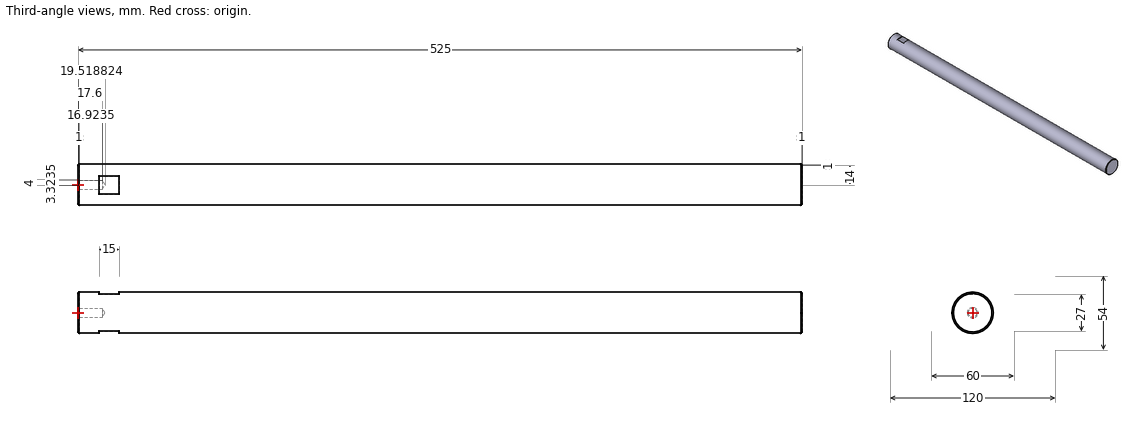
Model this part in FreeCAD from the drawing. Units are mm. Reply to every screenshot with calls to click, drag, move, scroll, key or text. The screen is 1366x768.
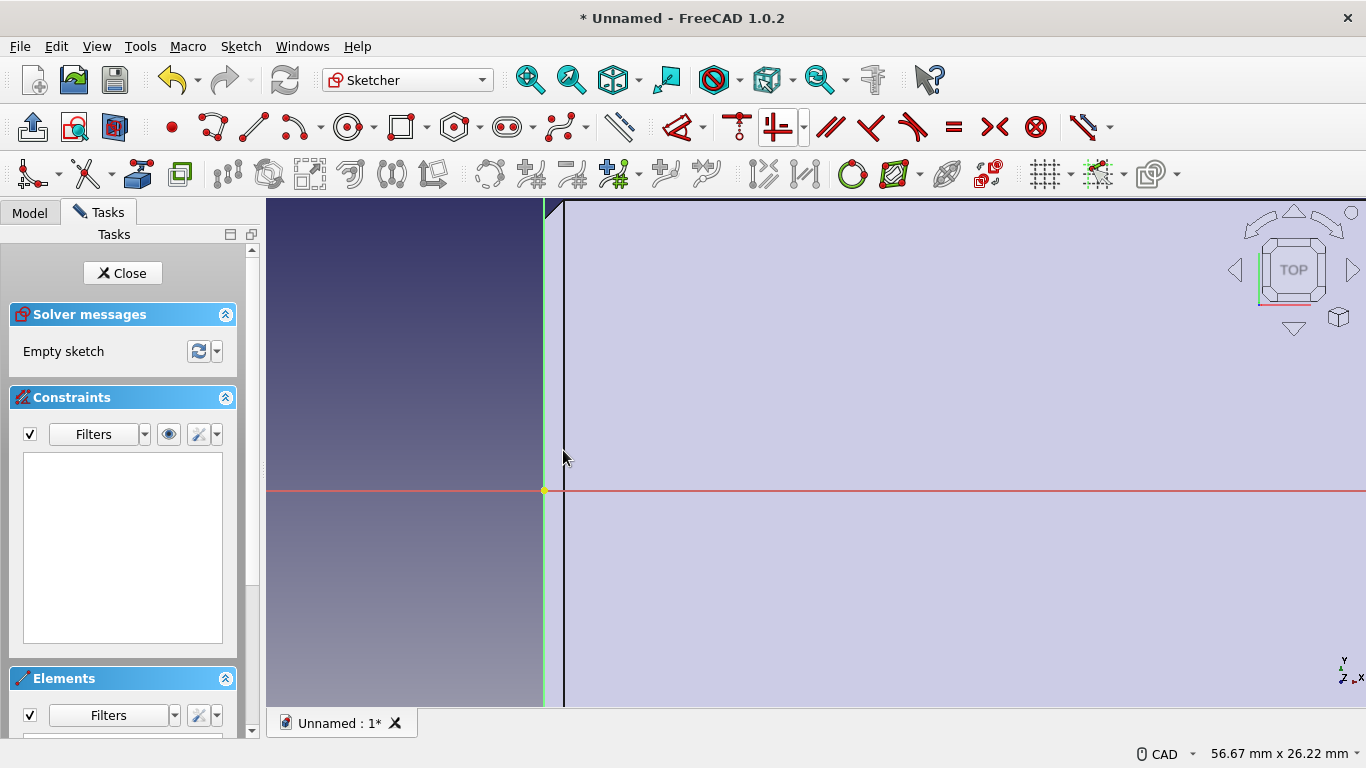
scroll(717, 451, up, 3)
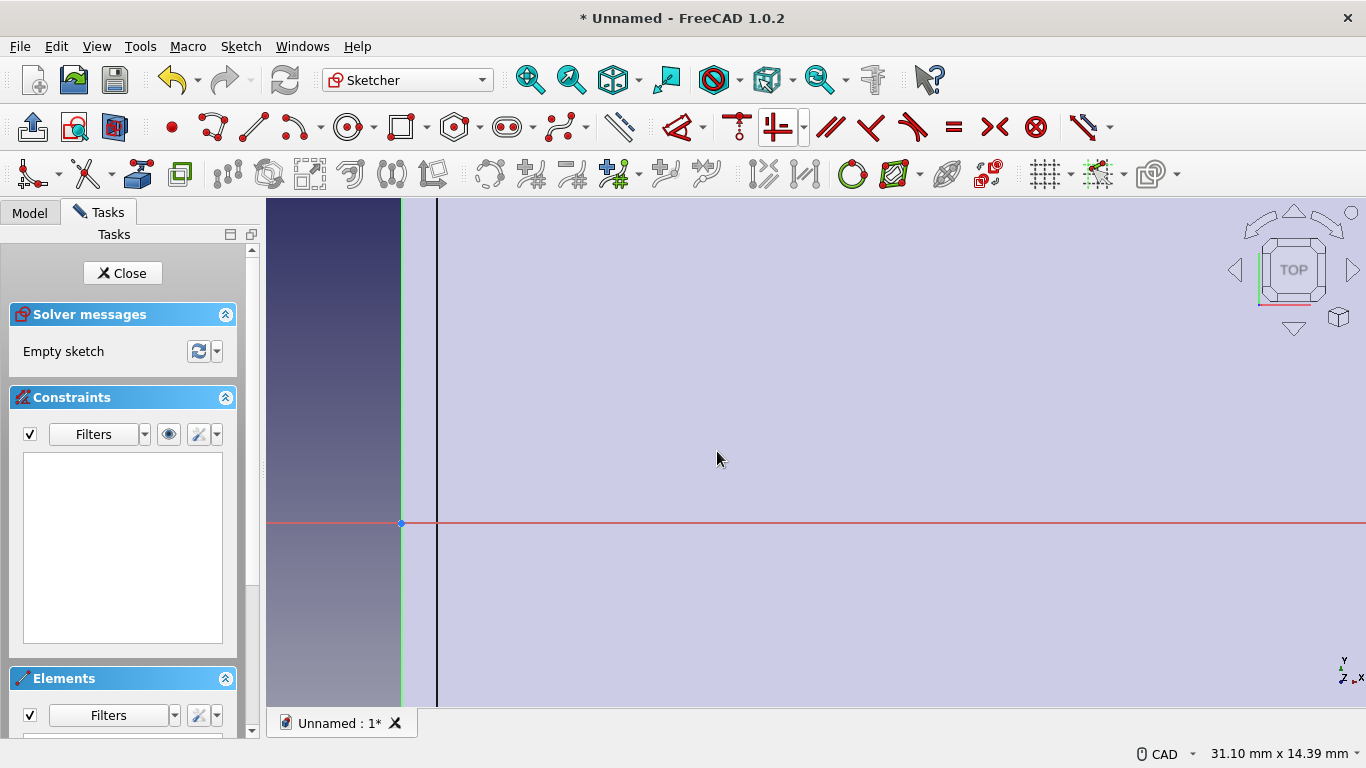
click(213, 128)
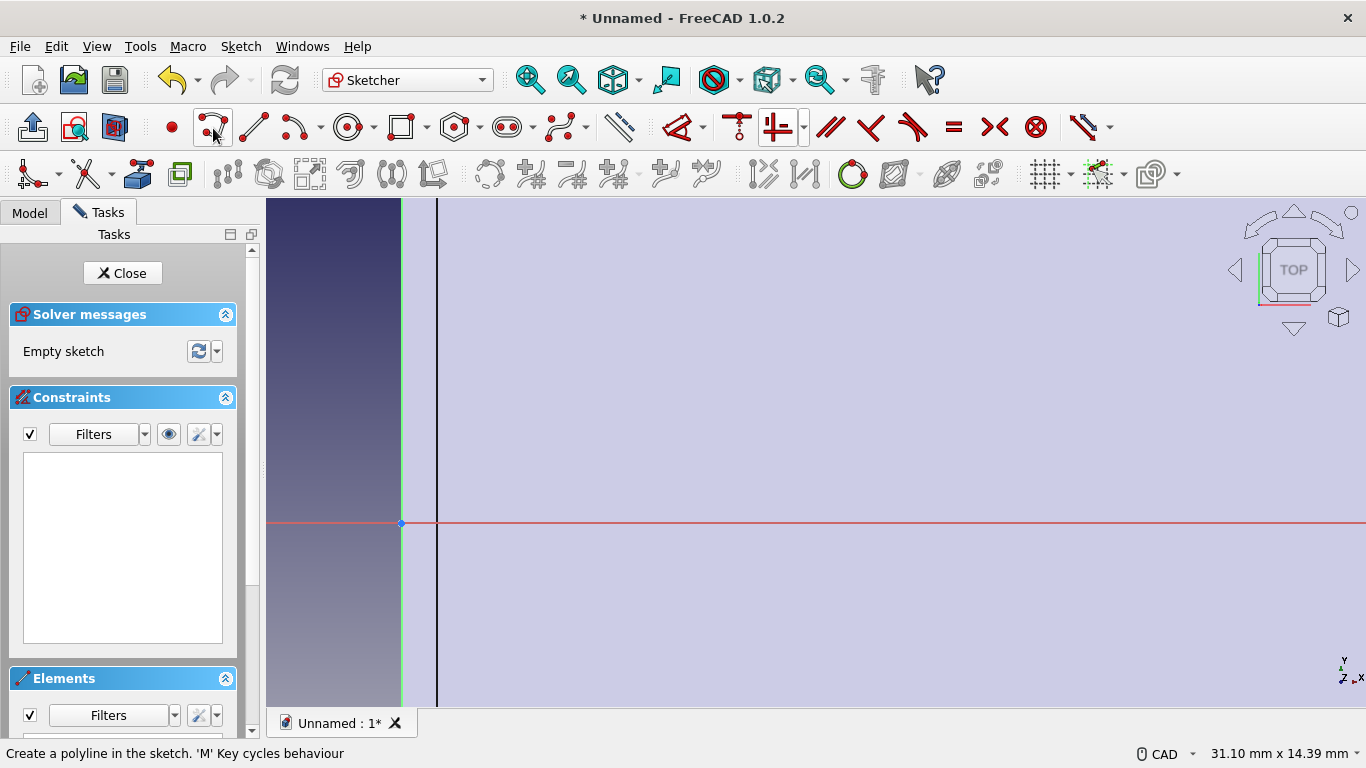
click(402, 523)
click(1092, 514)
click(1024, 405)
click(426, 405)
click(411, 382)
click(402, 523)
key(Escape)
key(Escape)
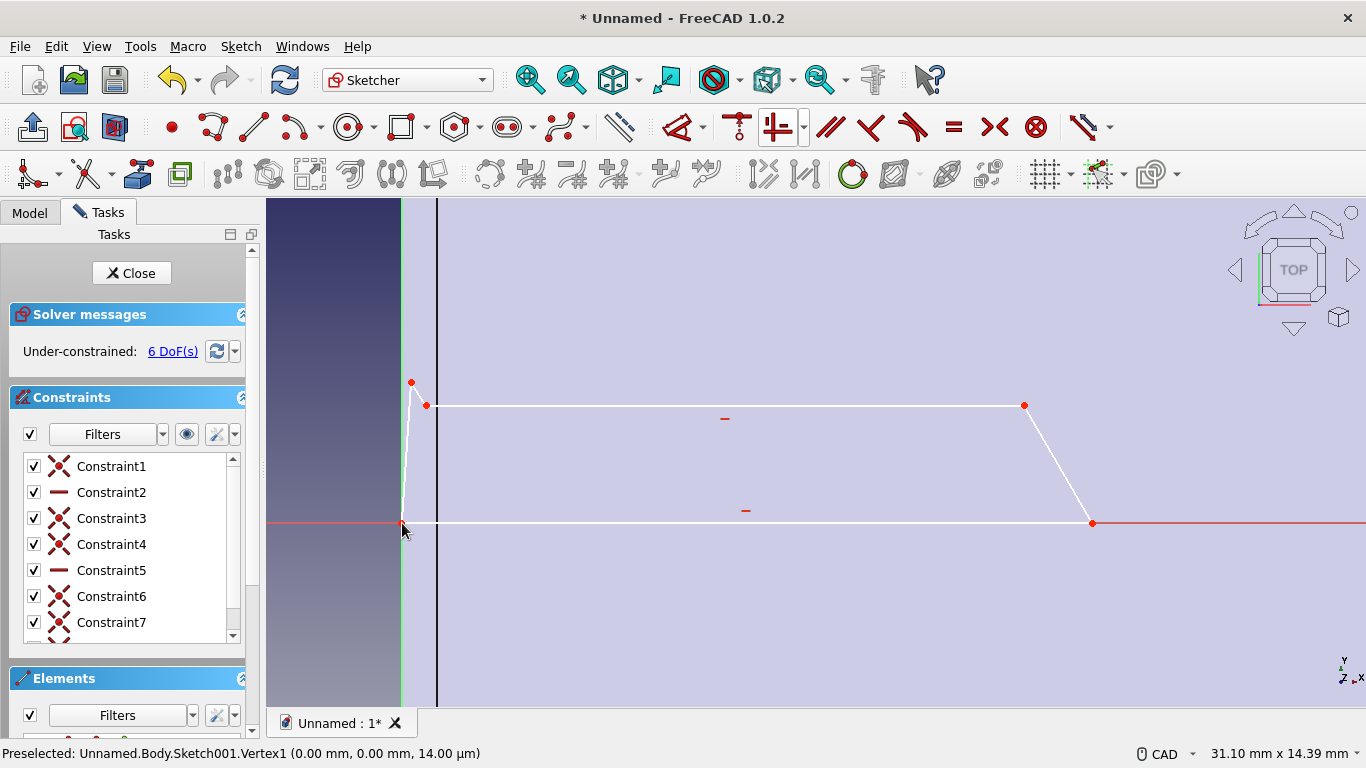
click(405, 481)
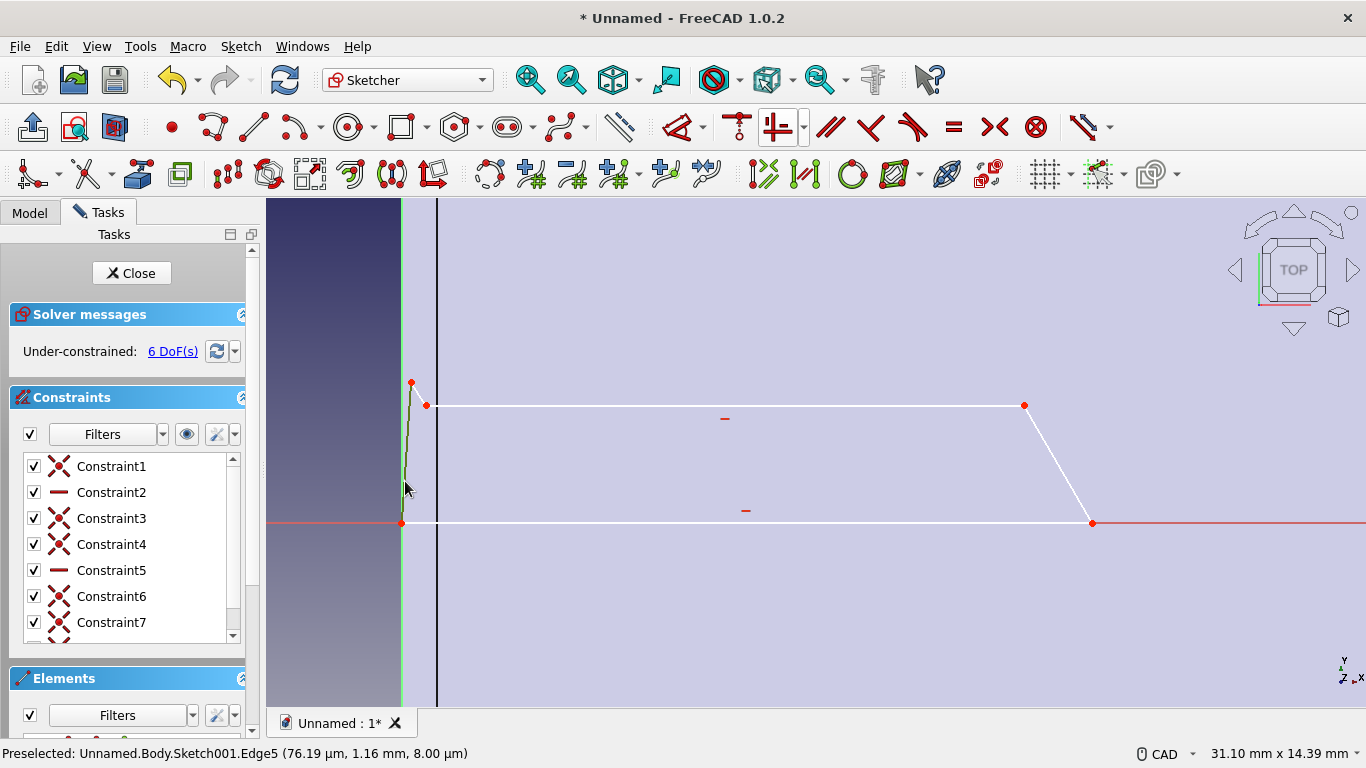
key(v)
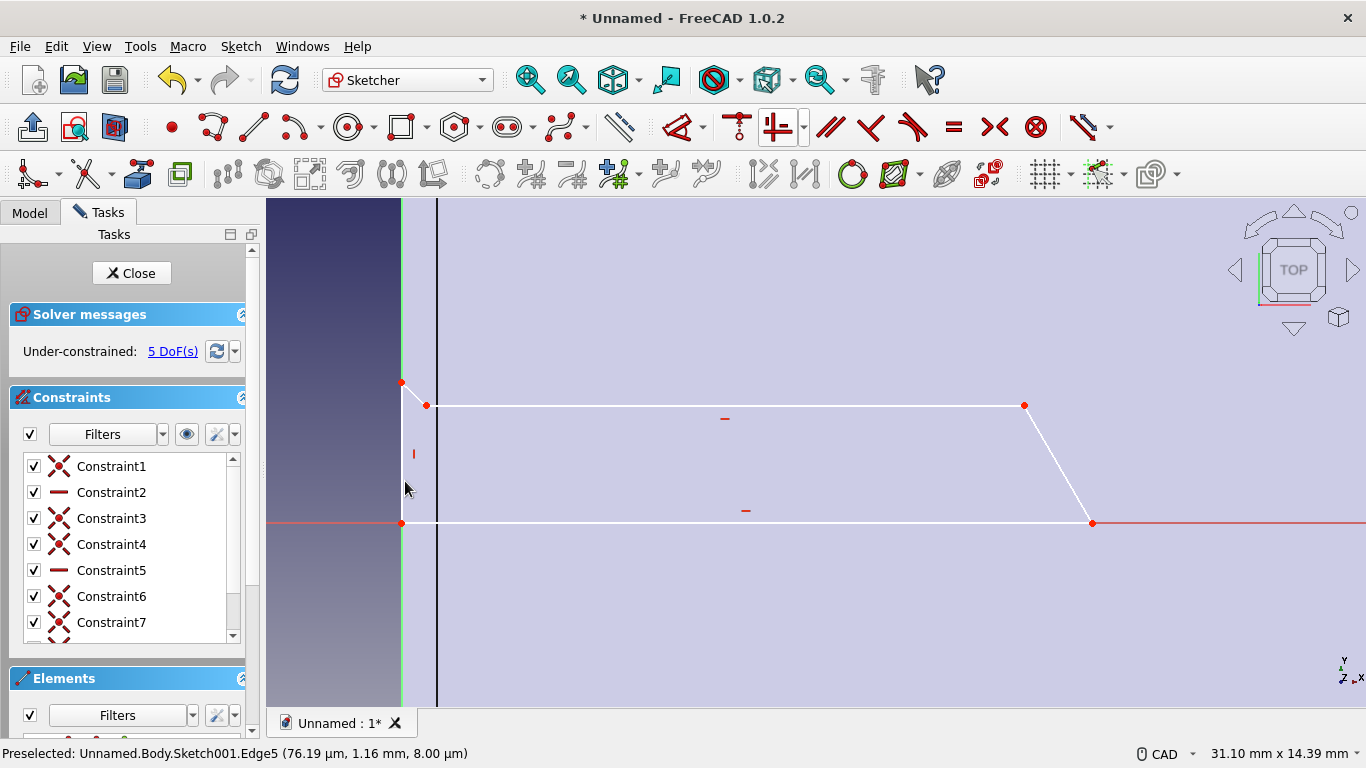
click(676, 128)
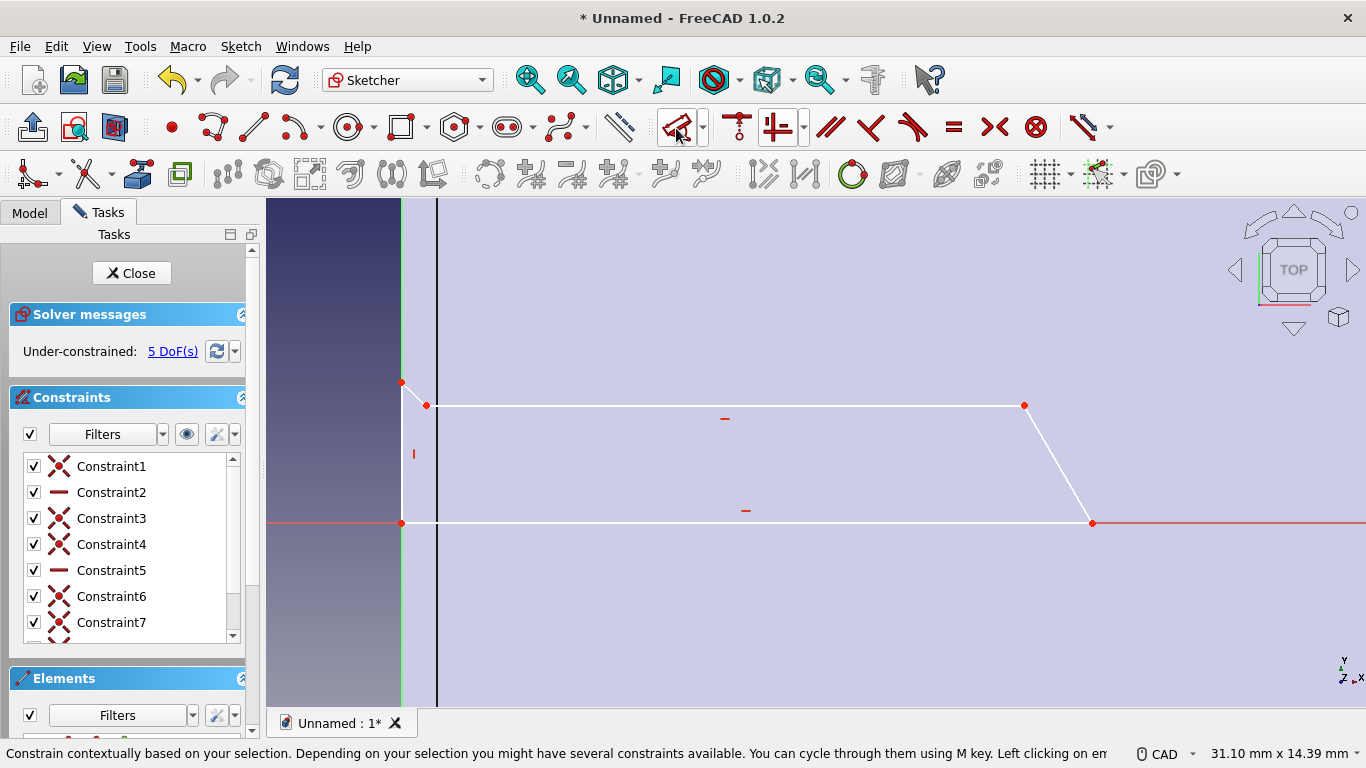
click(402, 425)
click(368, 453)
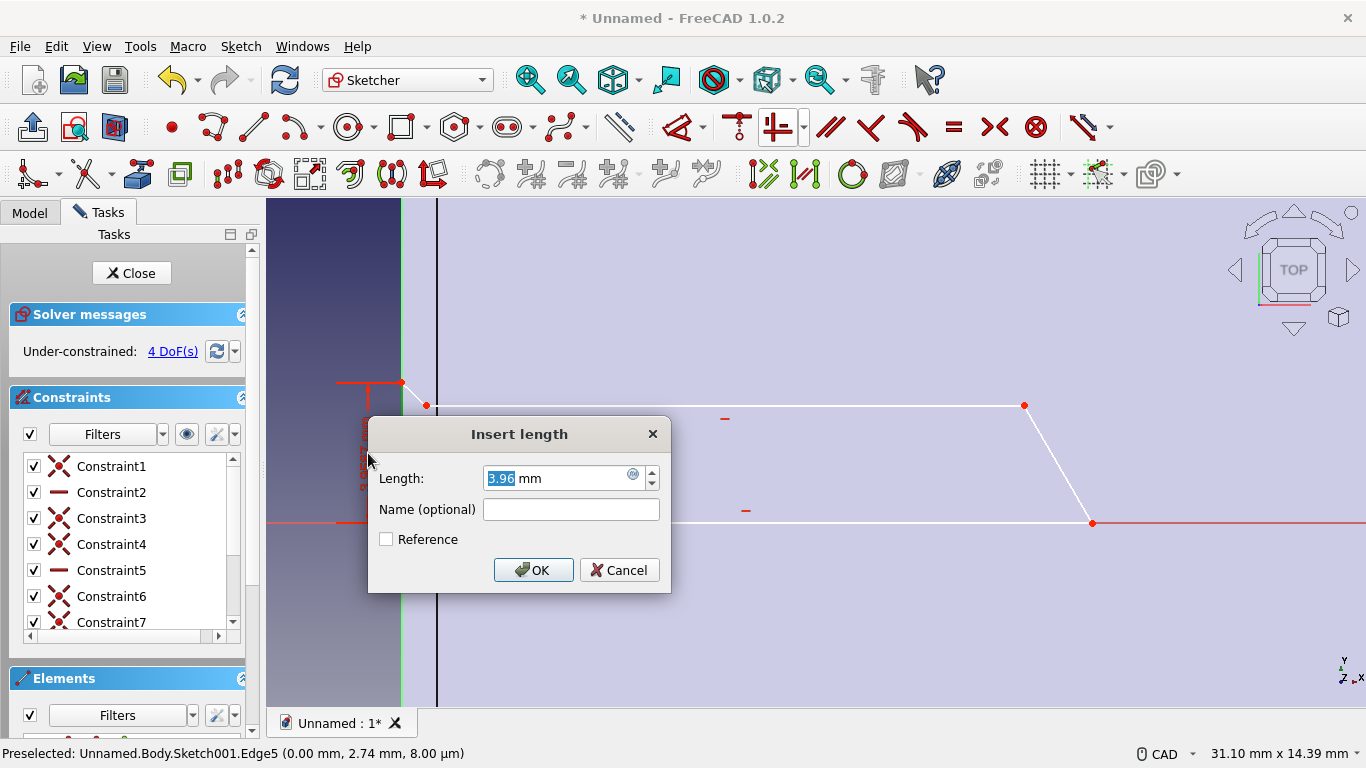
text(4)
key(Return)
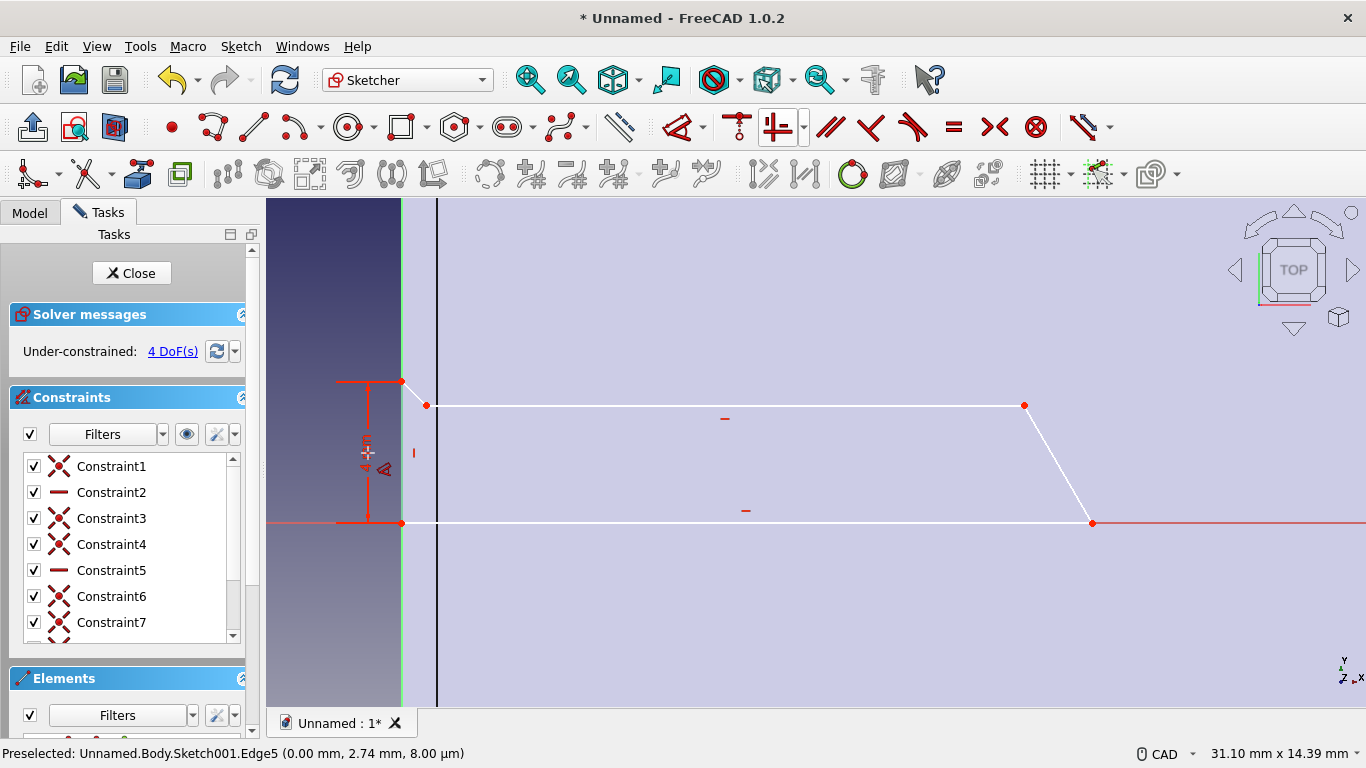
click(1024, 406)
click(713, 557)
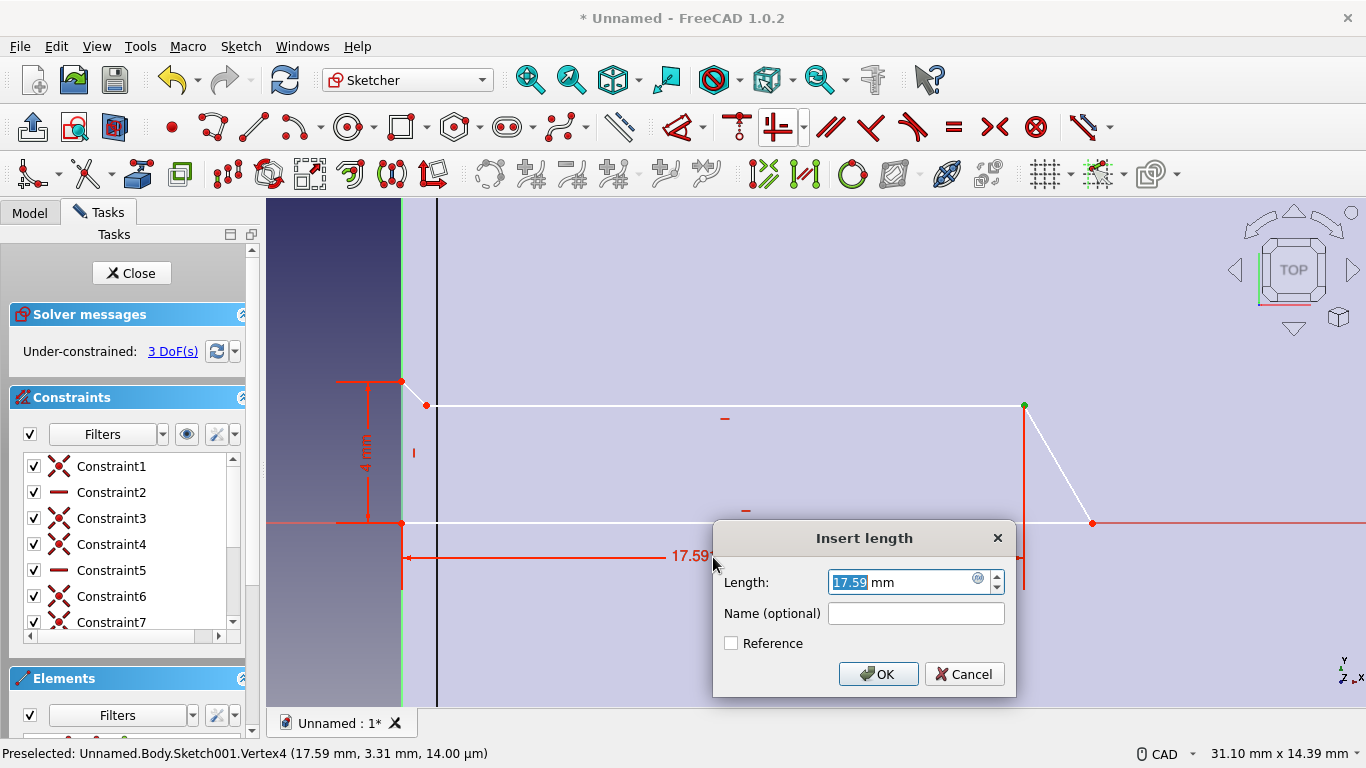
text(17.6)
key(Return)